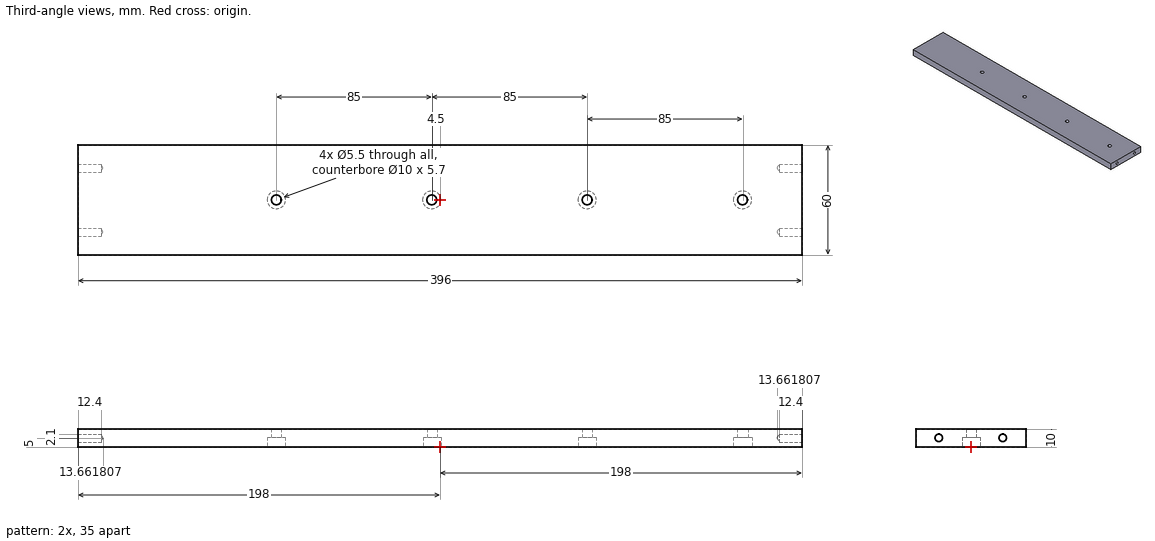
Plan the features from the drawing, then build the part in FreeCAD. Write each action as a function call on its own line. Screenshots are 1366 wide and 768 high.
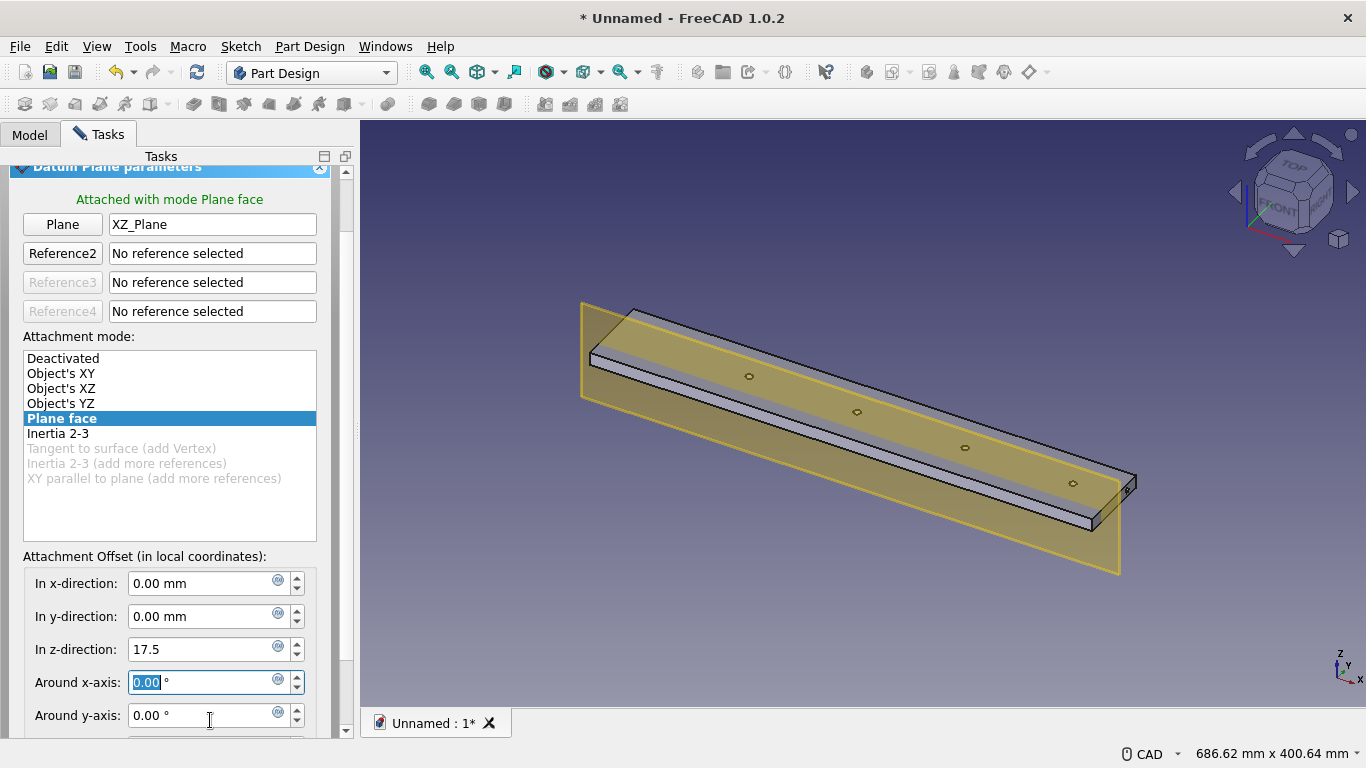
scroll(346, 452, up, 2)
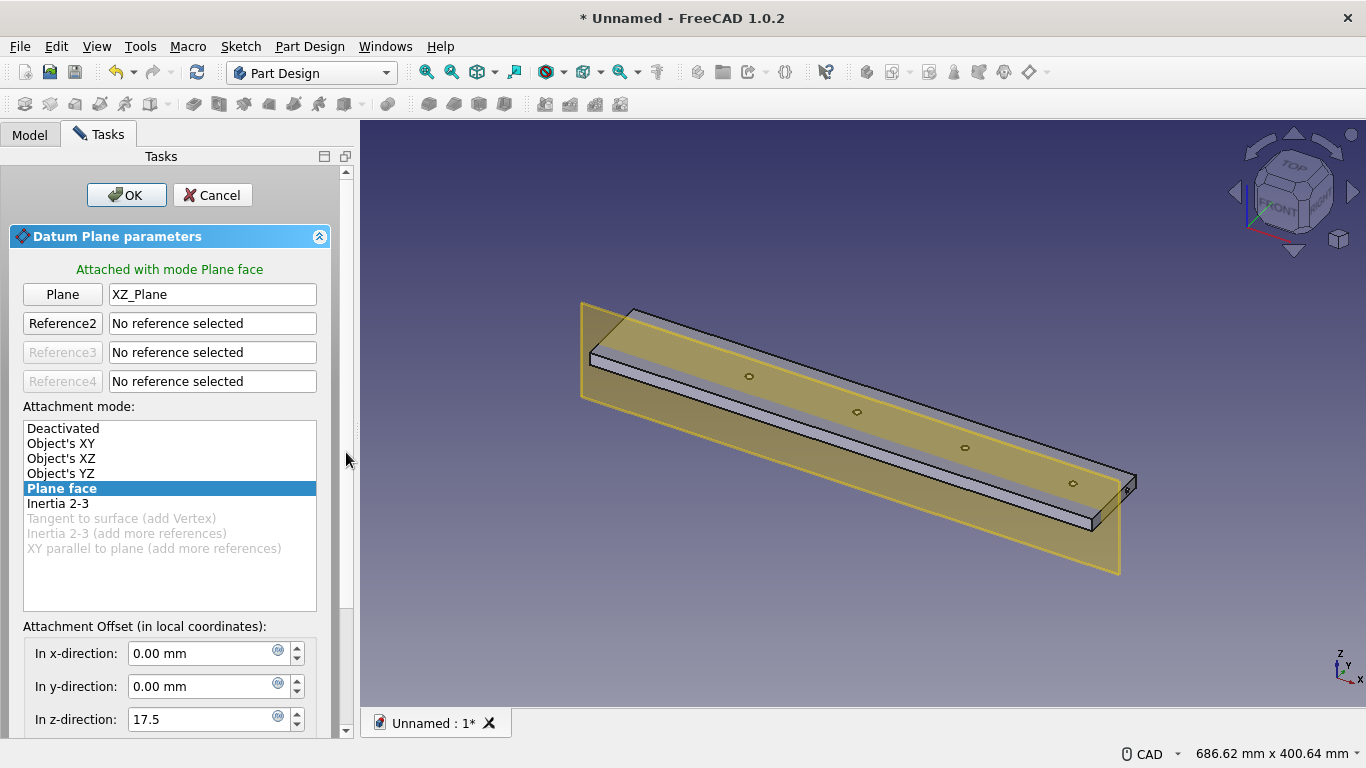
click(127, 195)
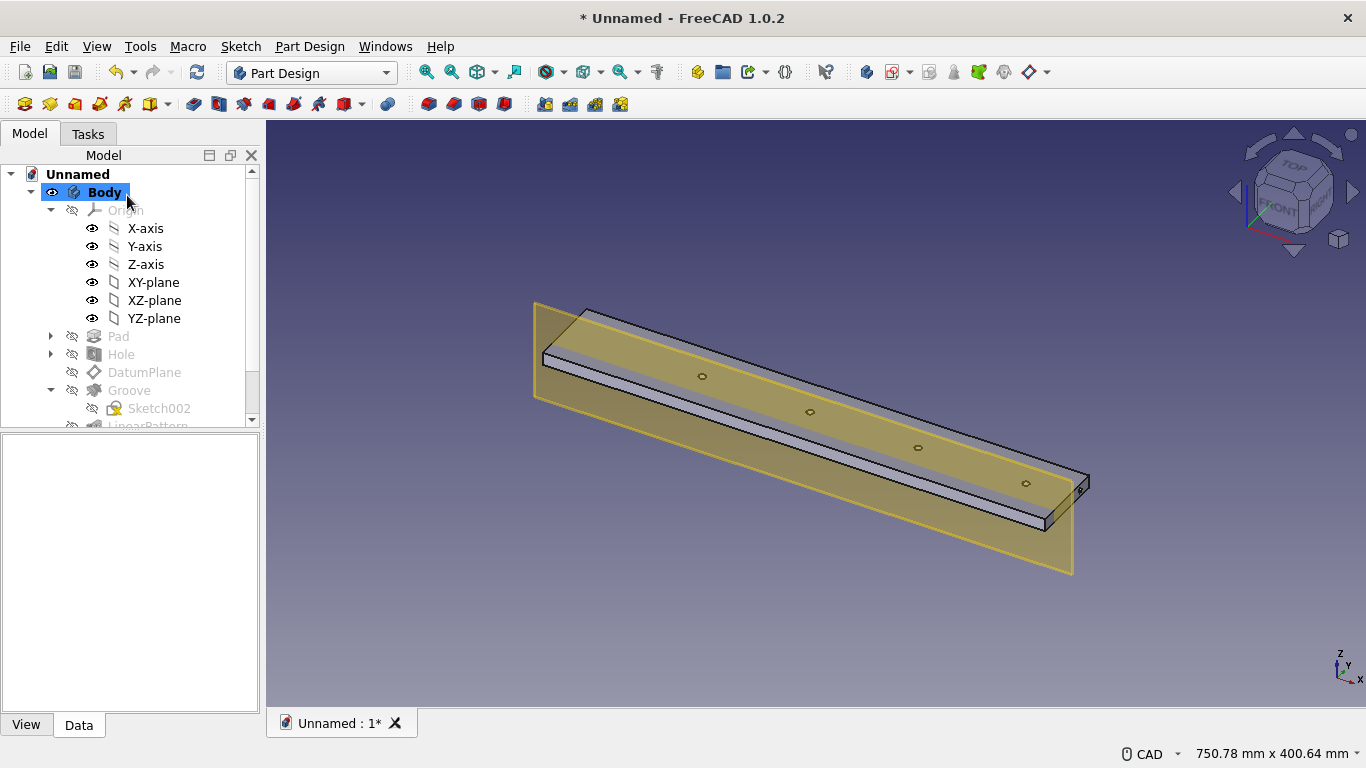
scroll(101, 296, down, 3)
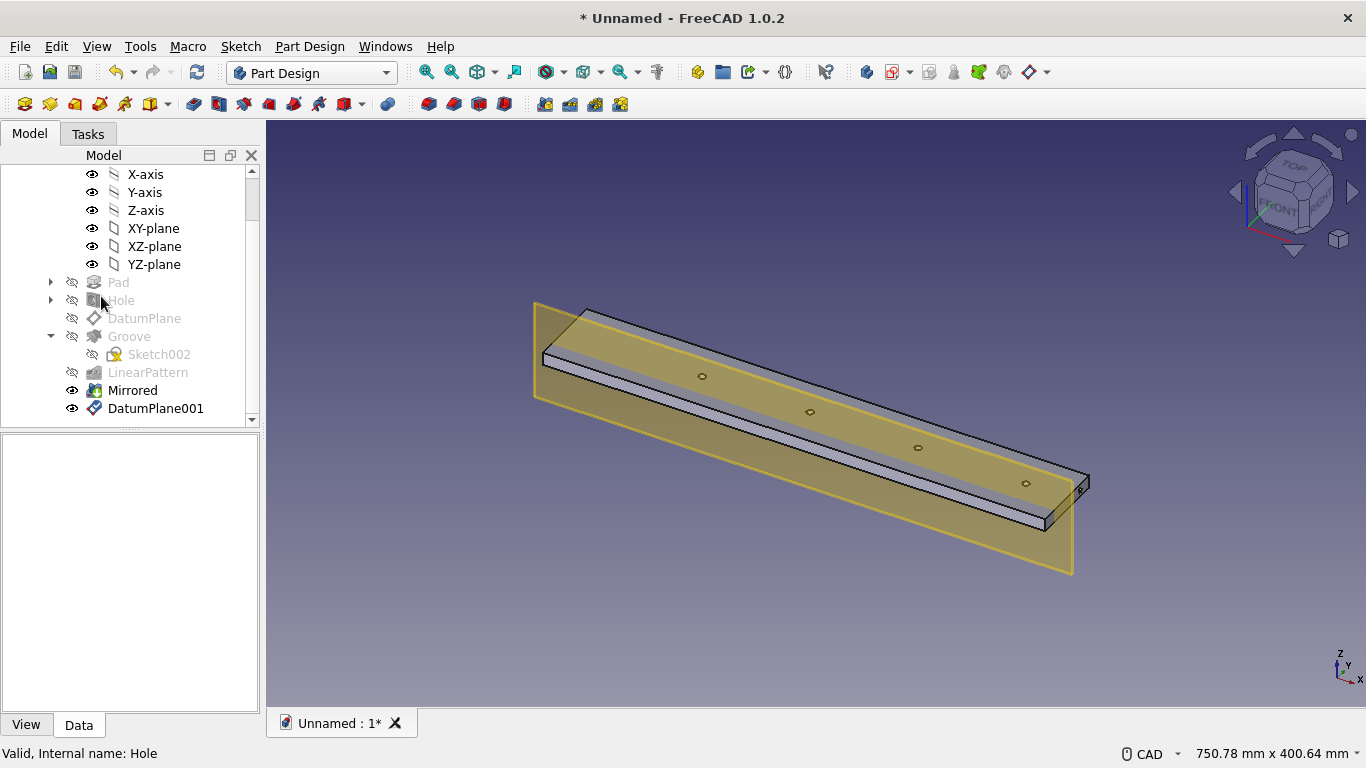
click(117, 408)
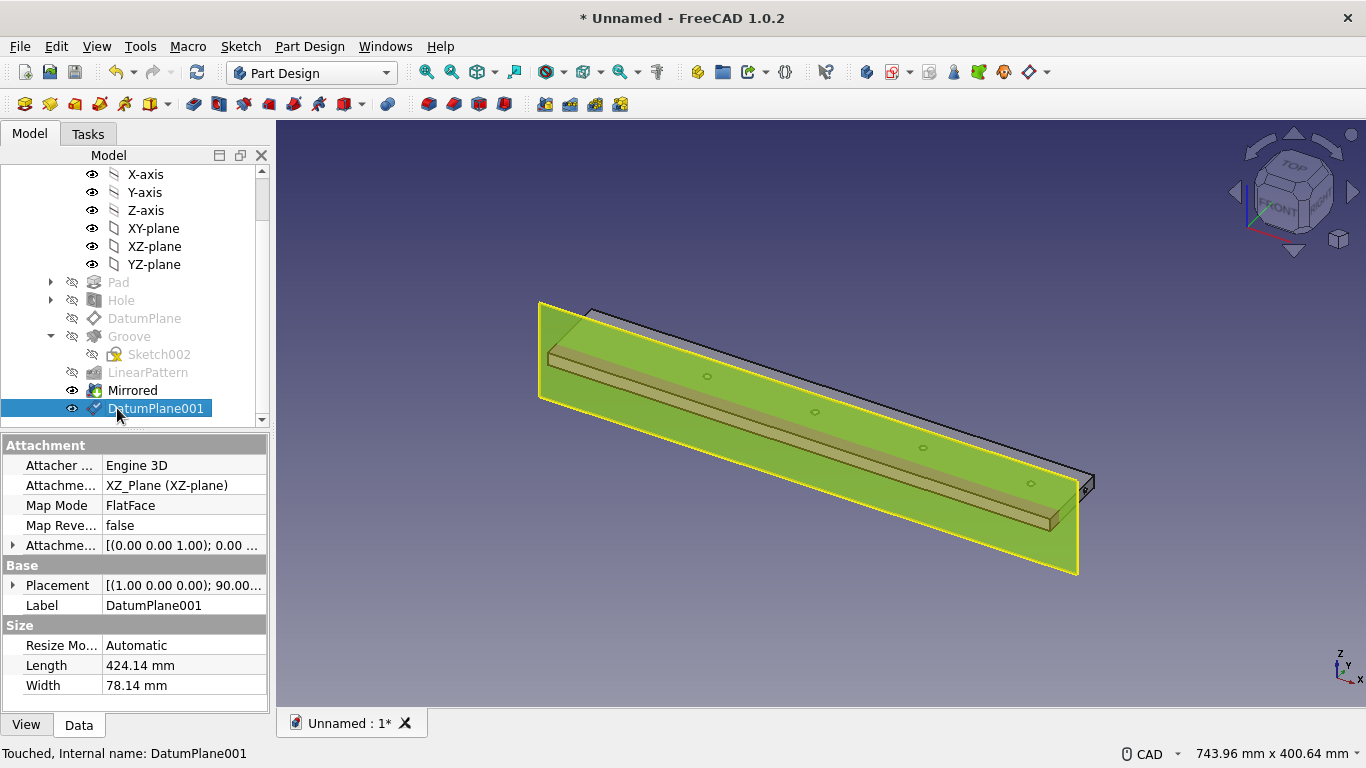
click(892, 72)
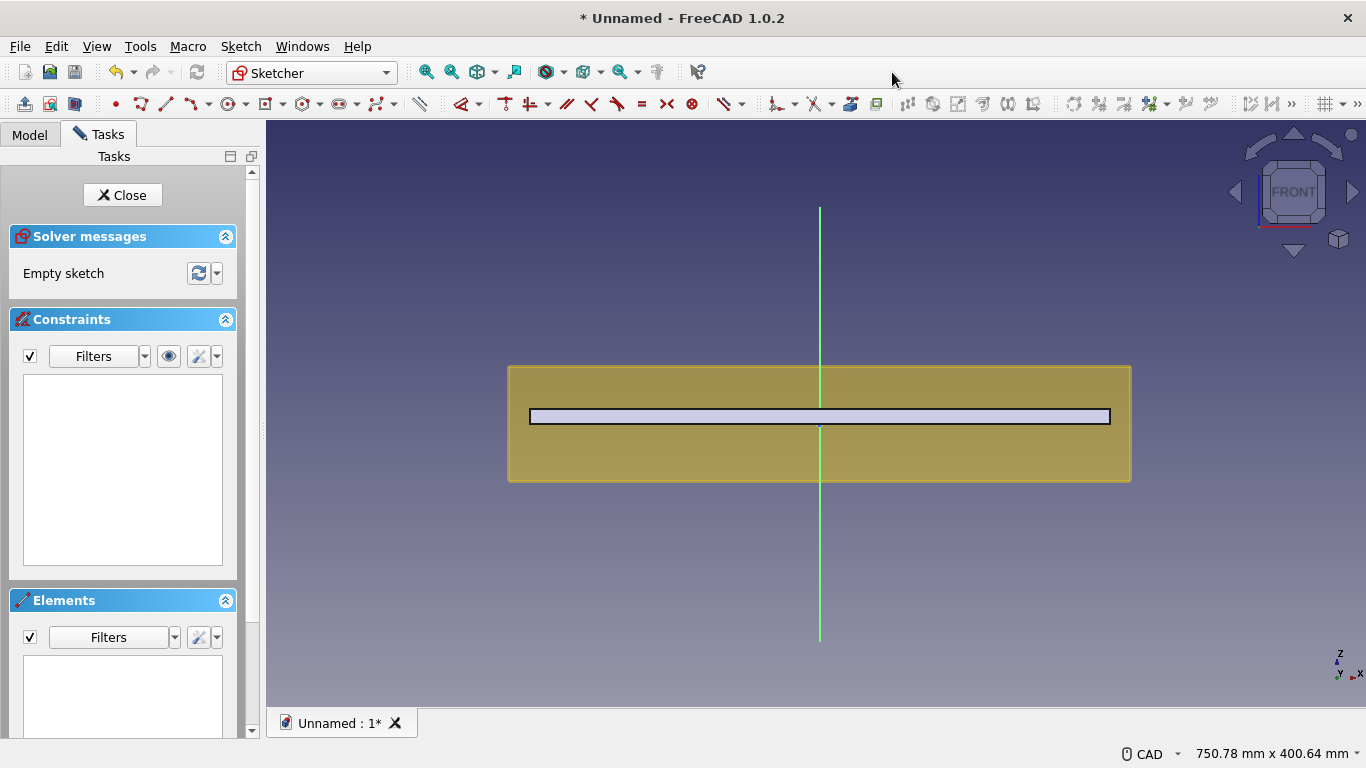
click(75, 104)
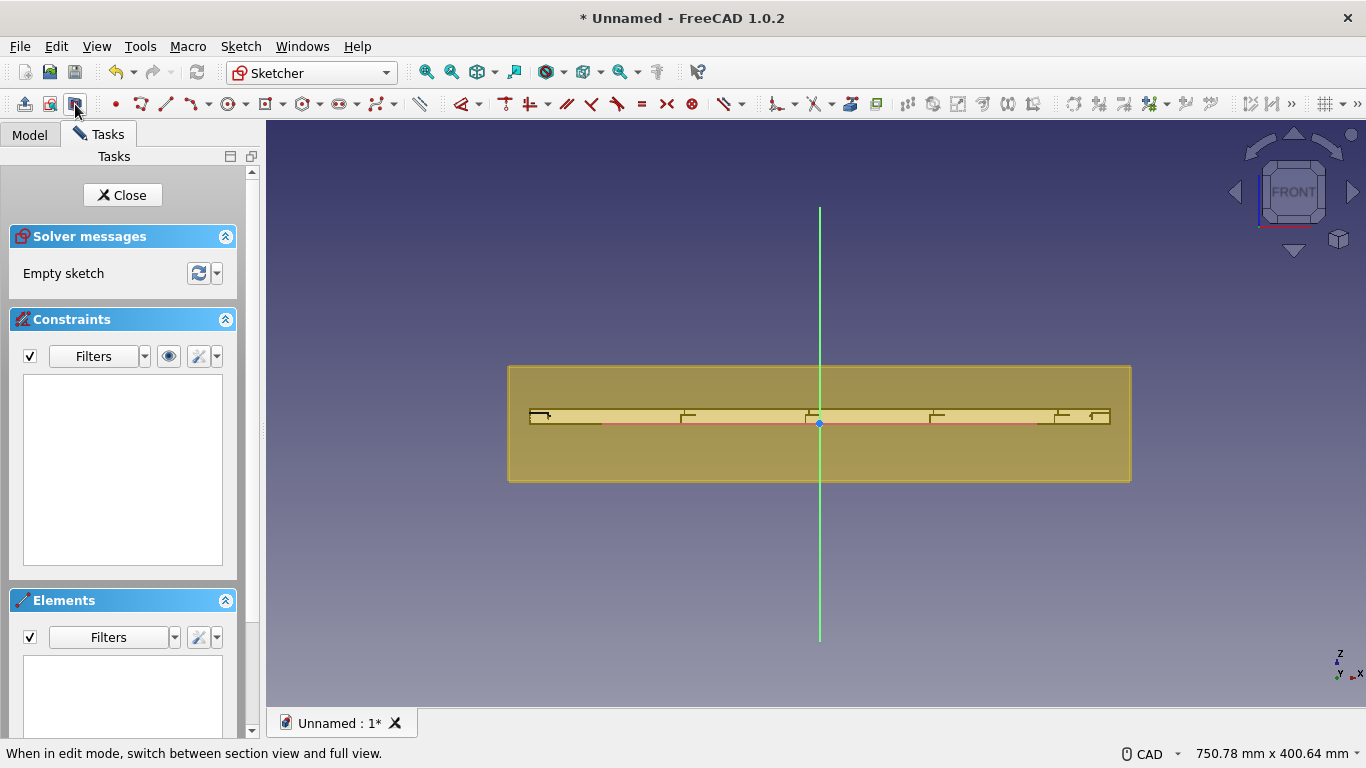
scroll(1122, 415, up, 15)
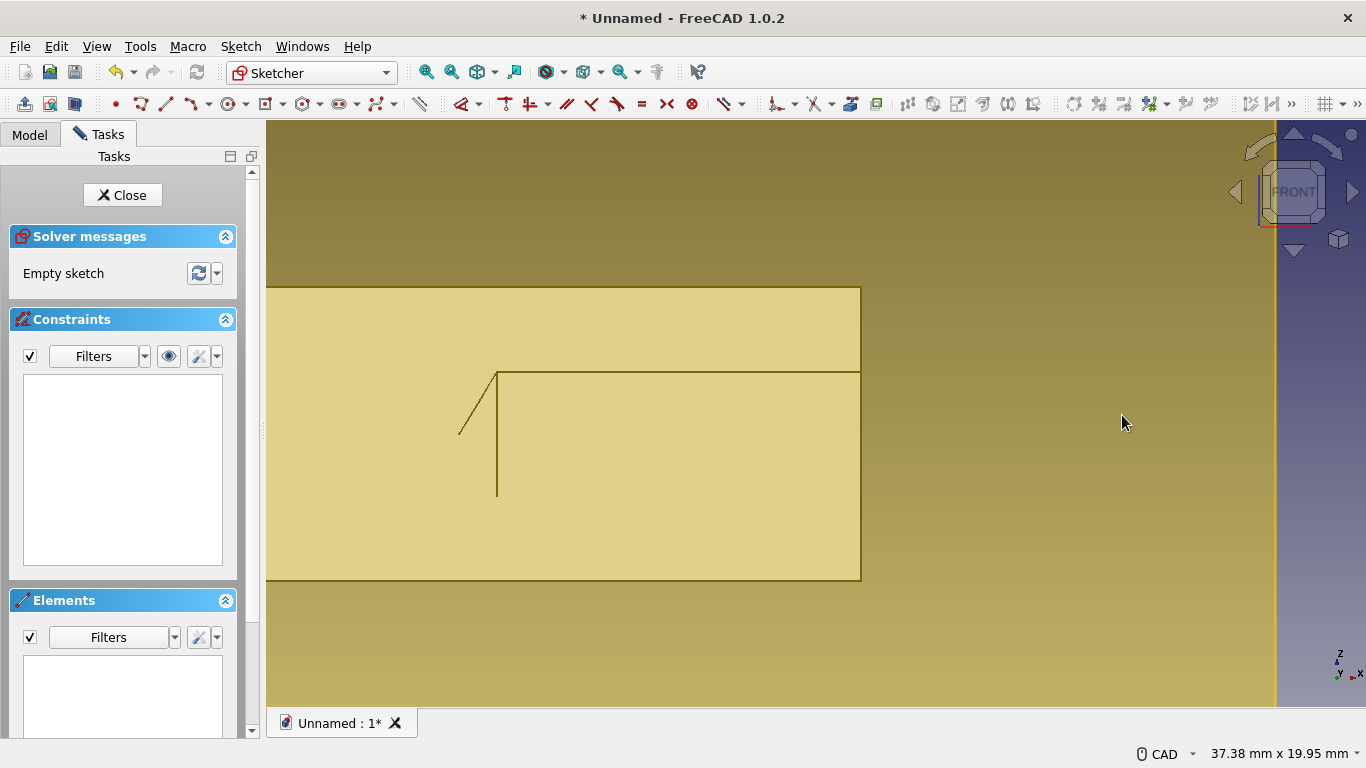
click(141, 104)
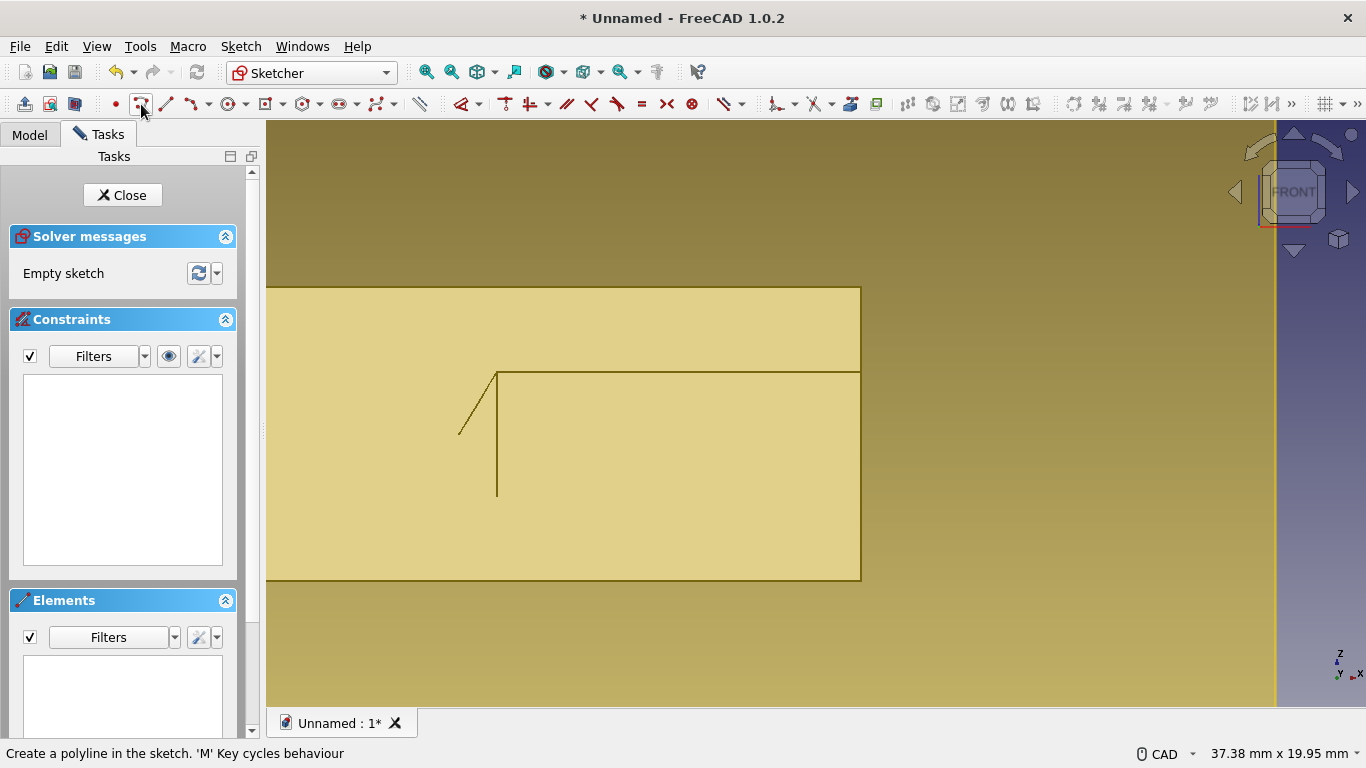
click(459, 434)
click(497, 372)
click(861, 372)
click(861, 434)
click(459, 435)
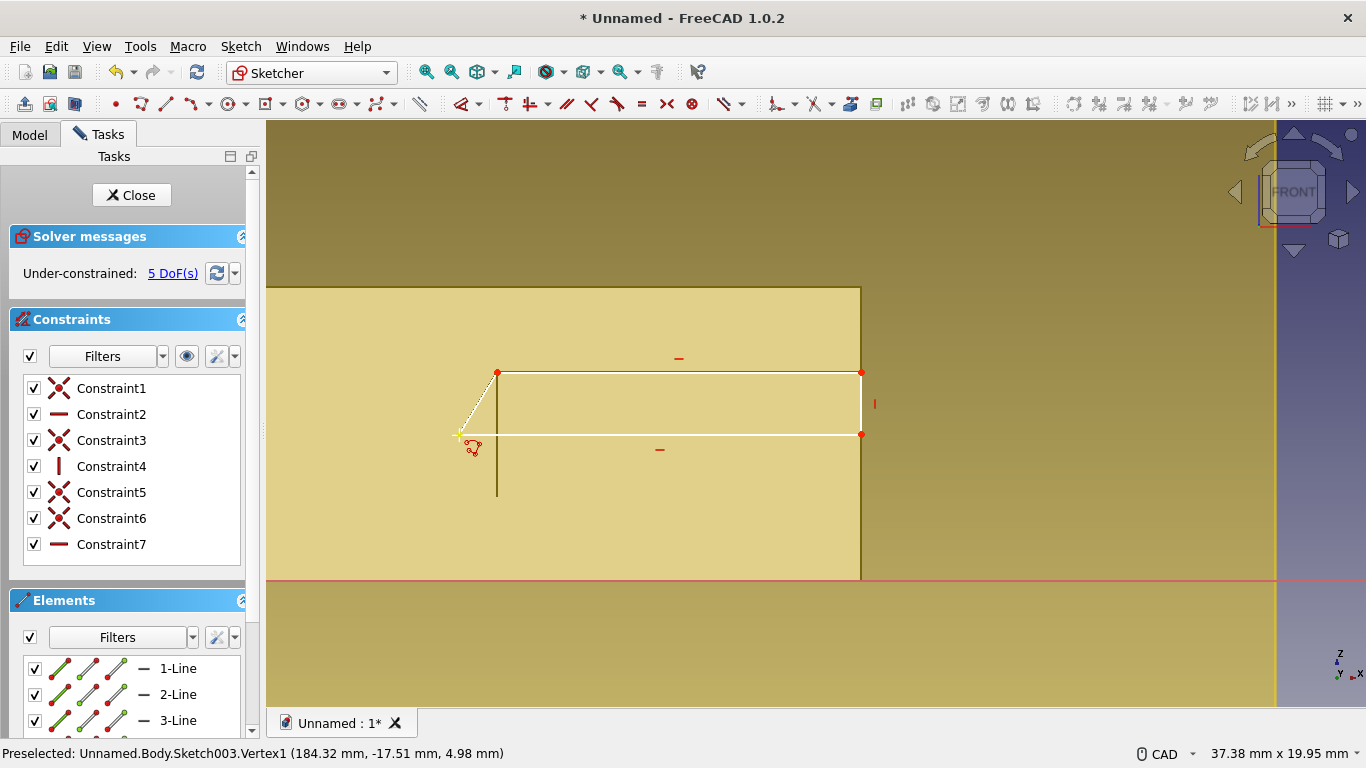
click(166, 104)